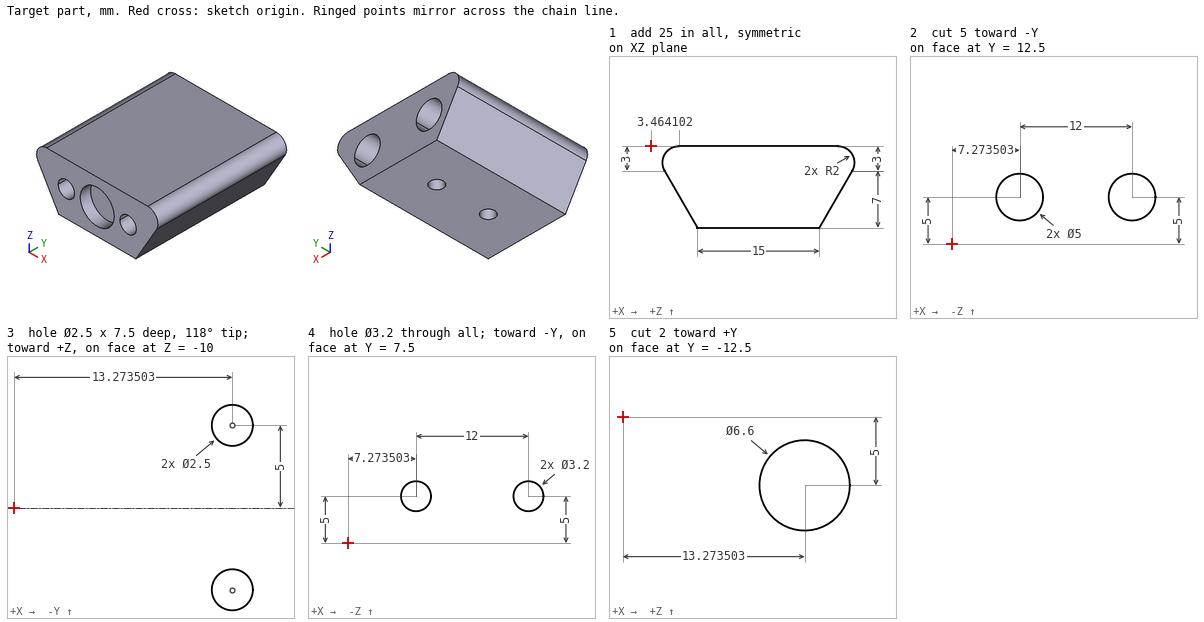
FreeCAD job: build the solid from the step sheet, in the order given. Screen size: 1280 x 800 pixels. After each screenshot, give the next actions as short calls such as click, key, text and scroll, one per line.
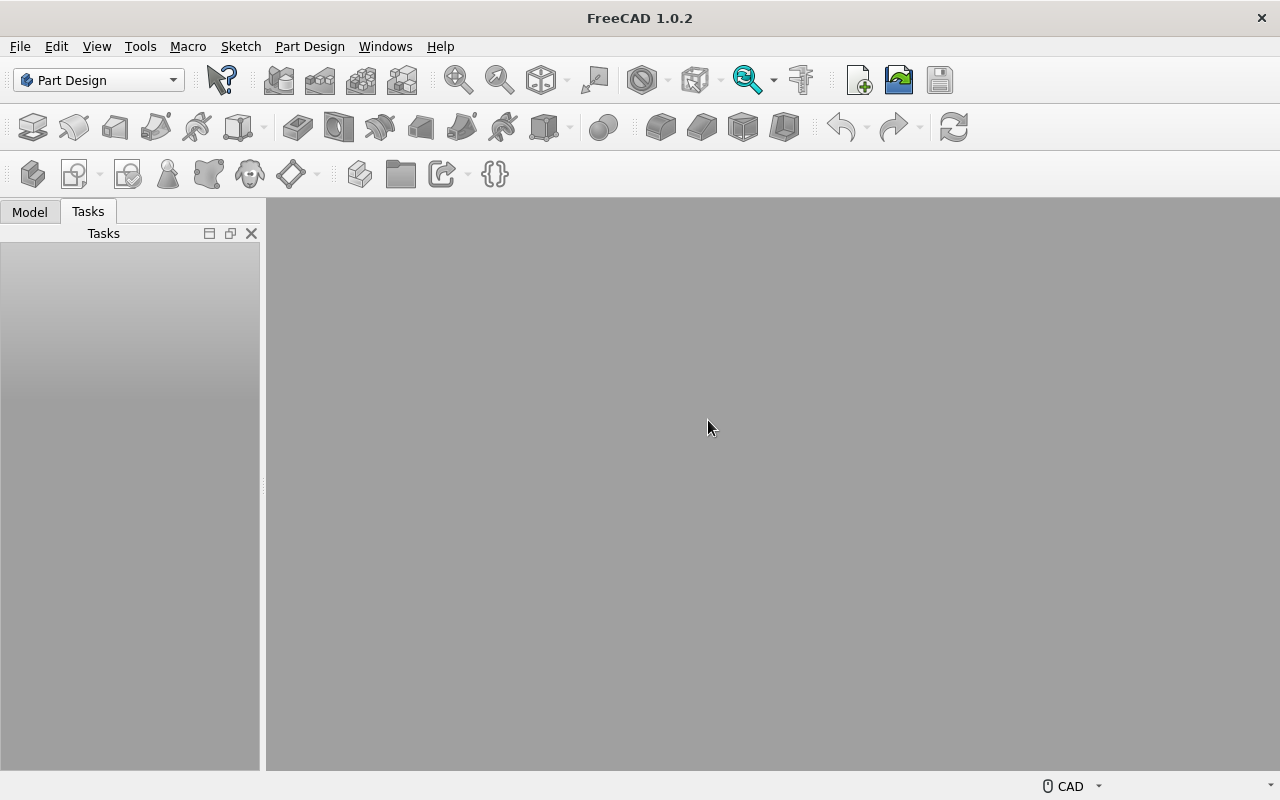
click(858, 80)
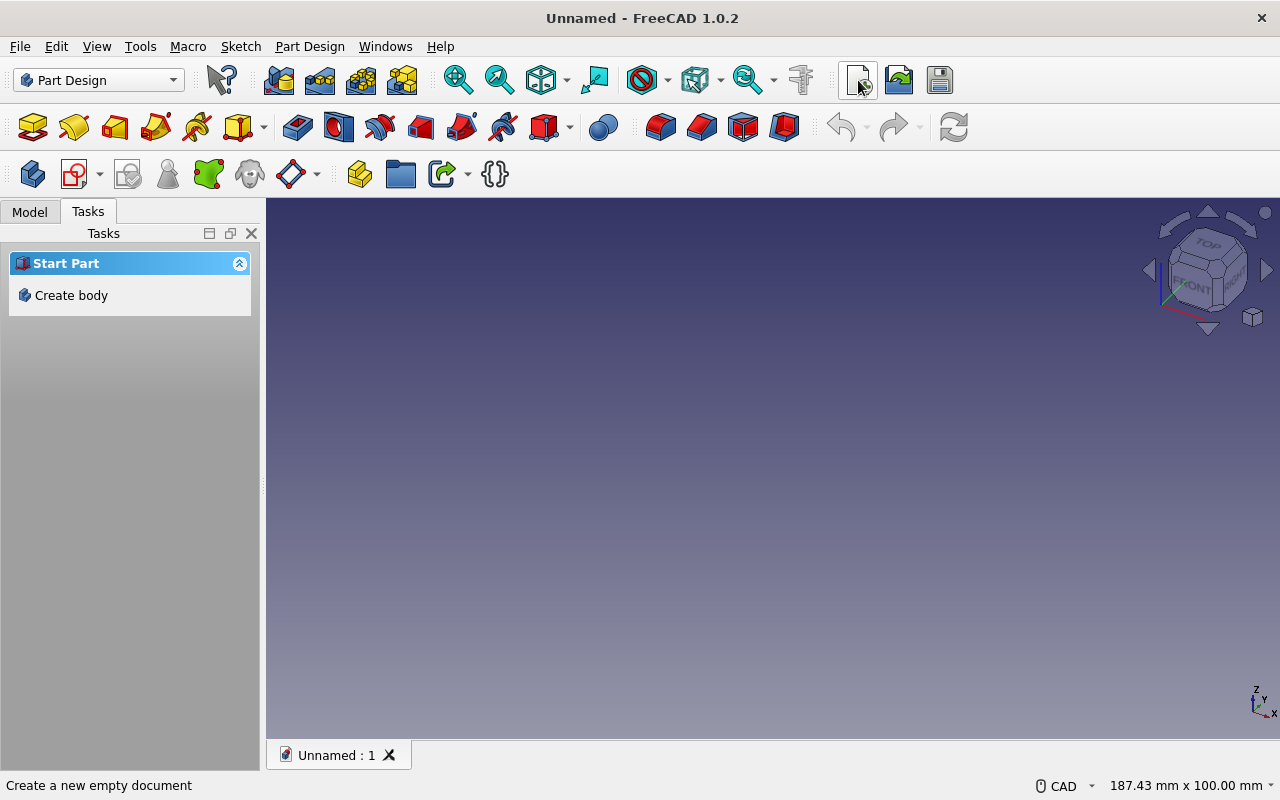
click(74, 174)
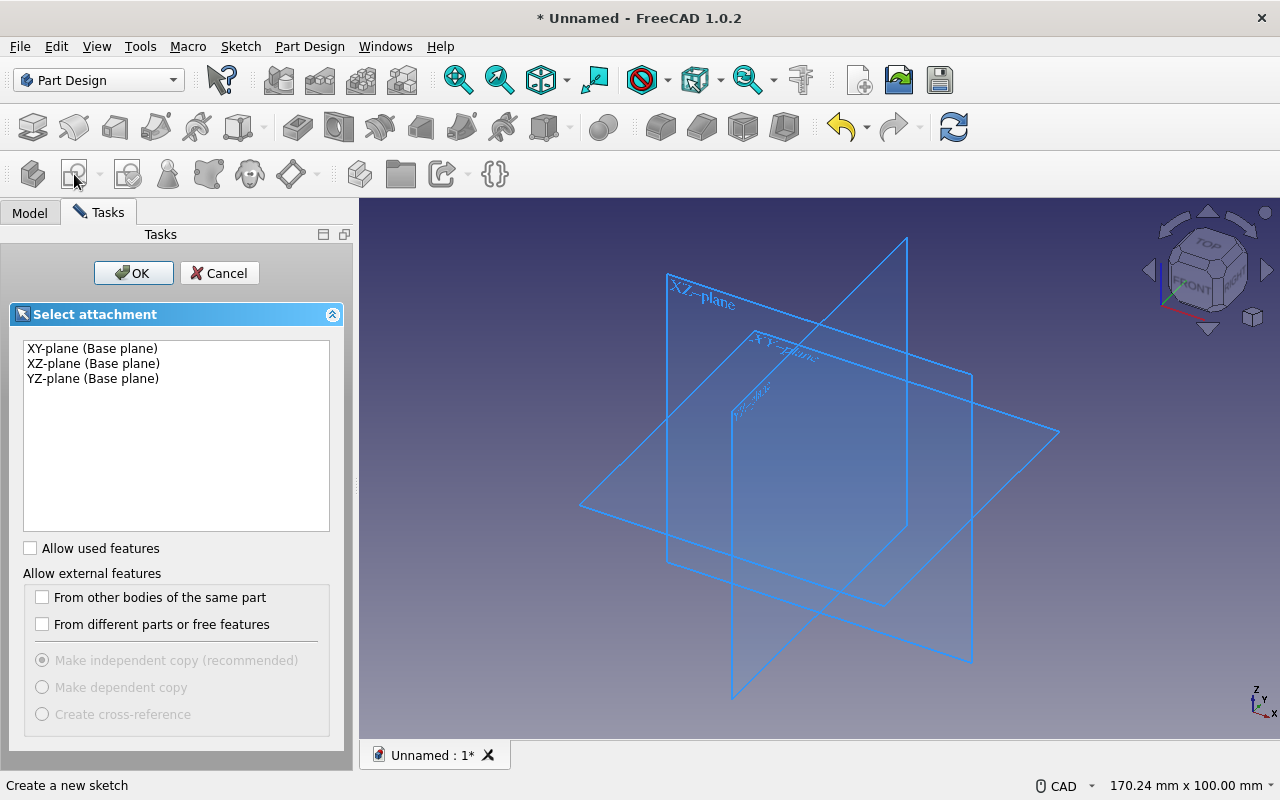
click(84, 364)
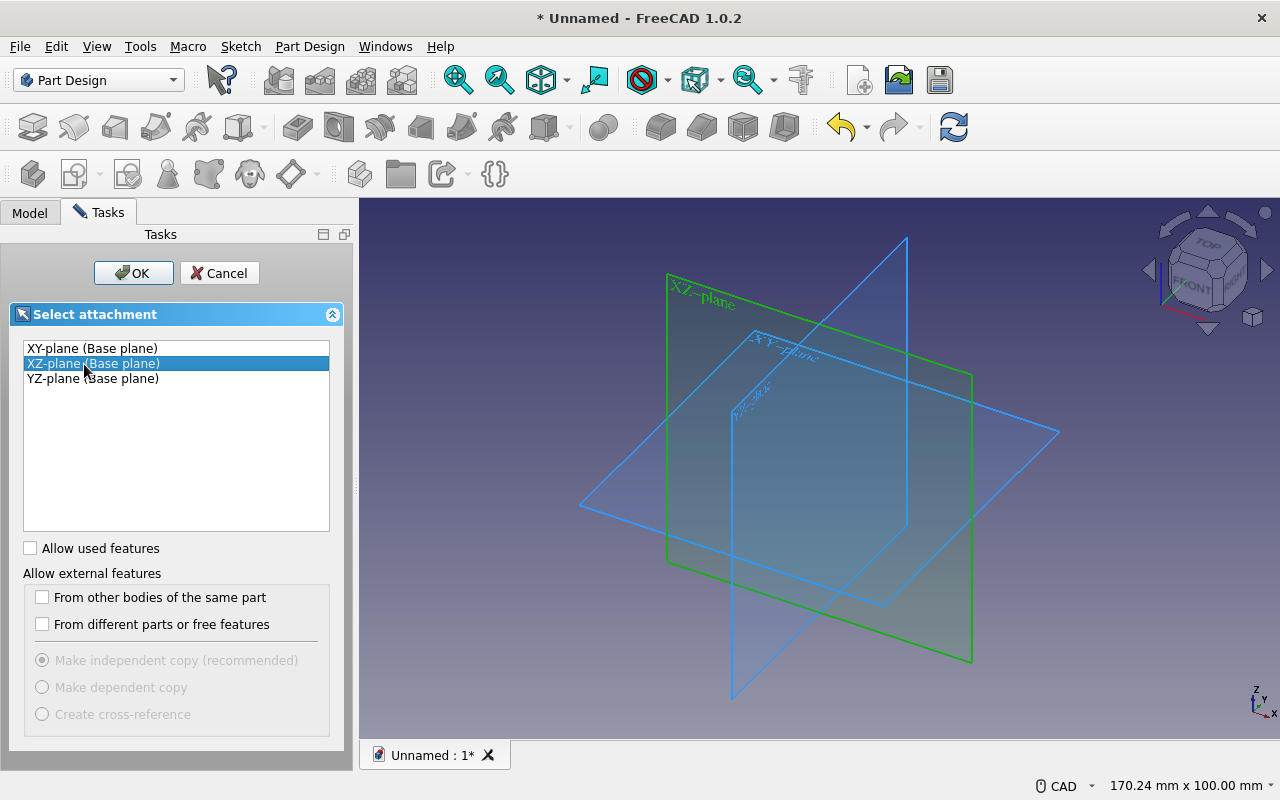
click(134, 273)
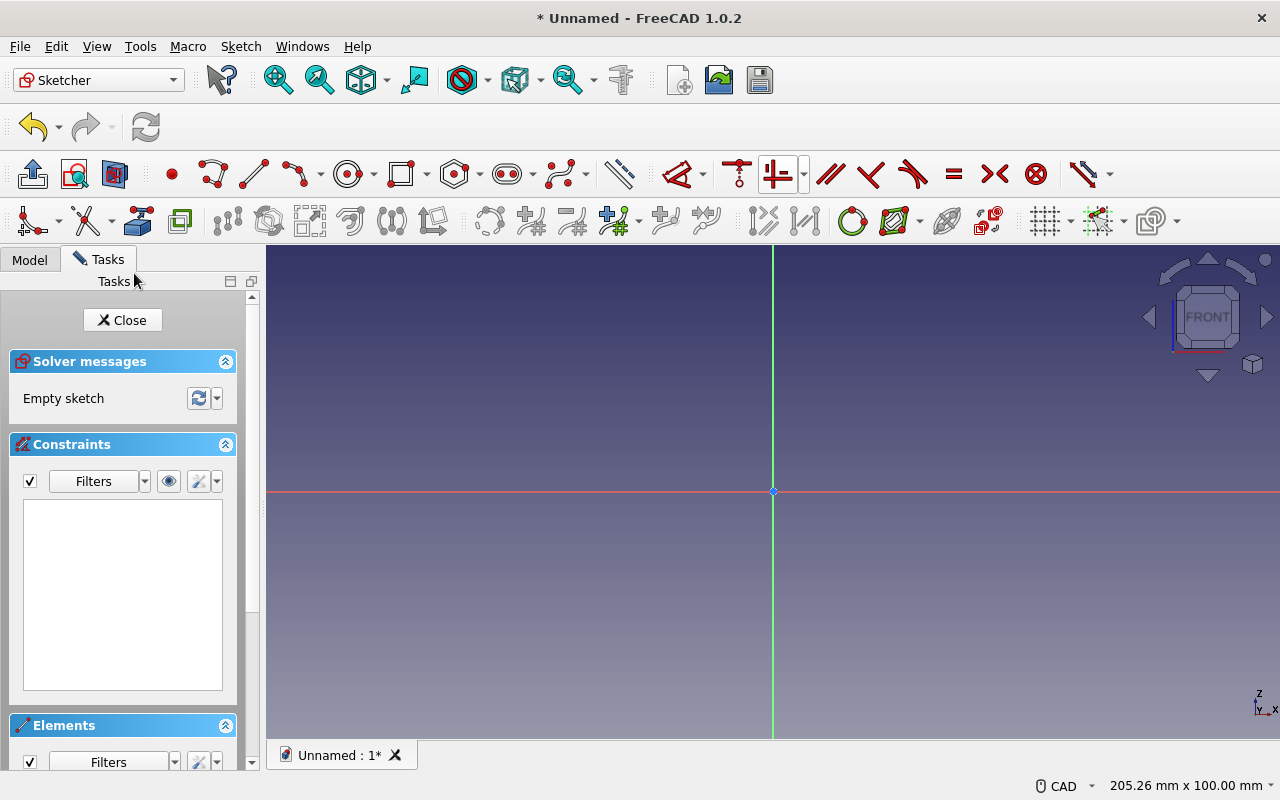
scroll(867, 523, up, 8)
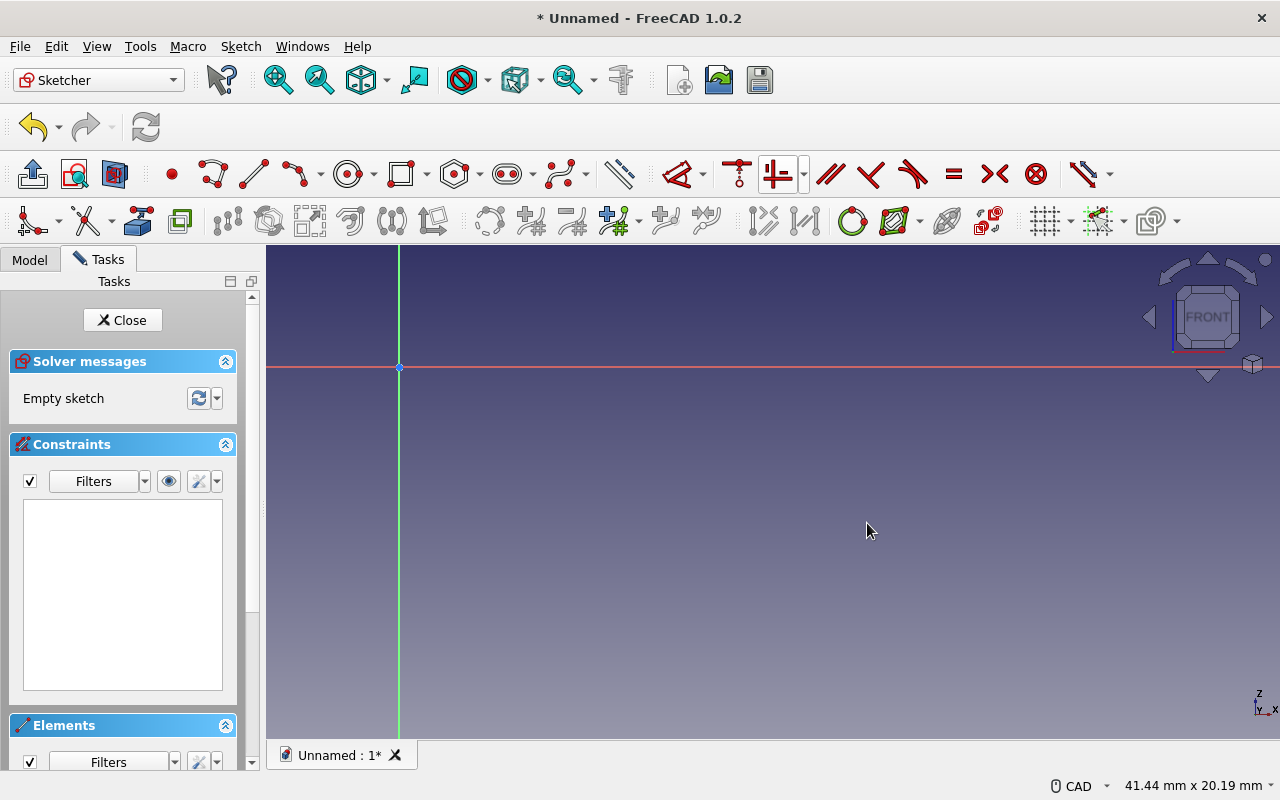
click(254, 174)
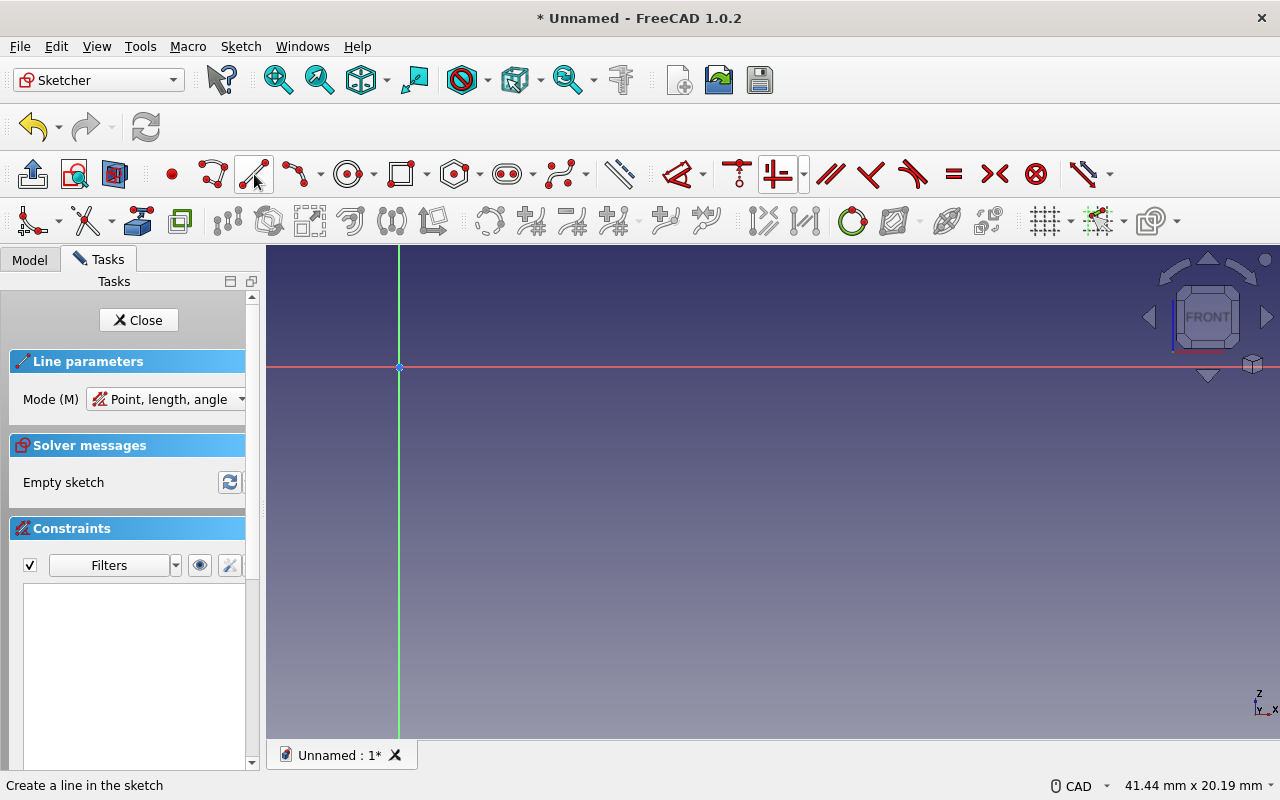
click(484, 367)
click(964, 376)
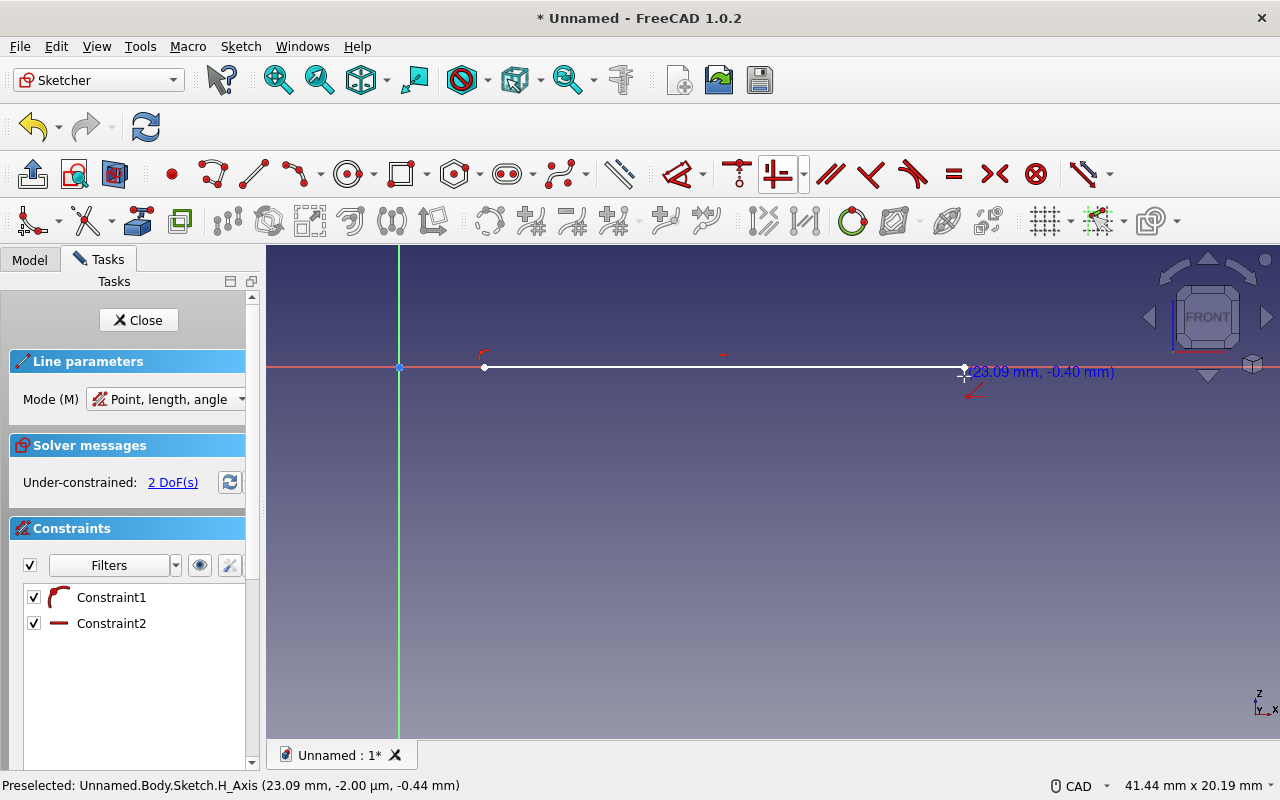
click(213, 174)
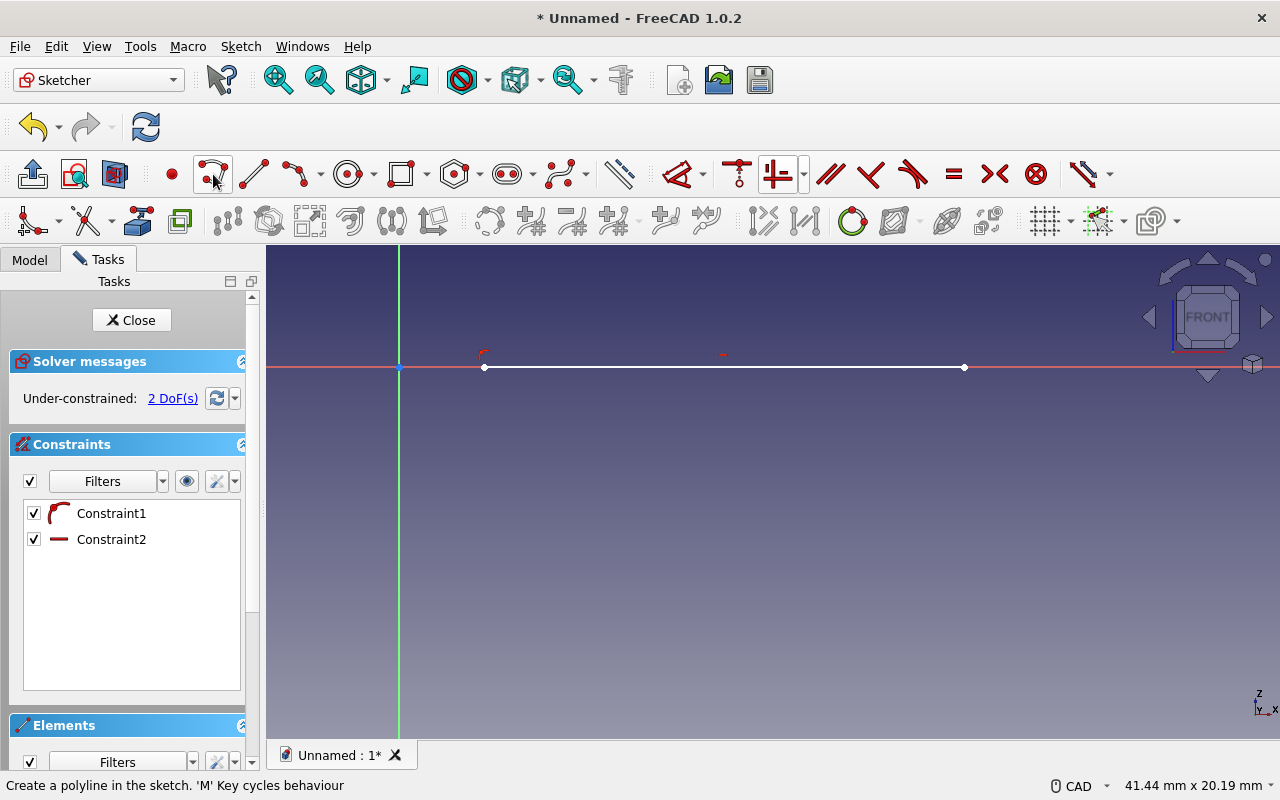
click(1006, 441)
click(907, 612)
click(540, 612)
click(441, 441)
right_click(441, 441)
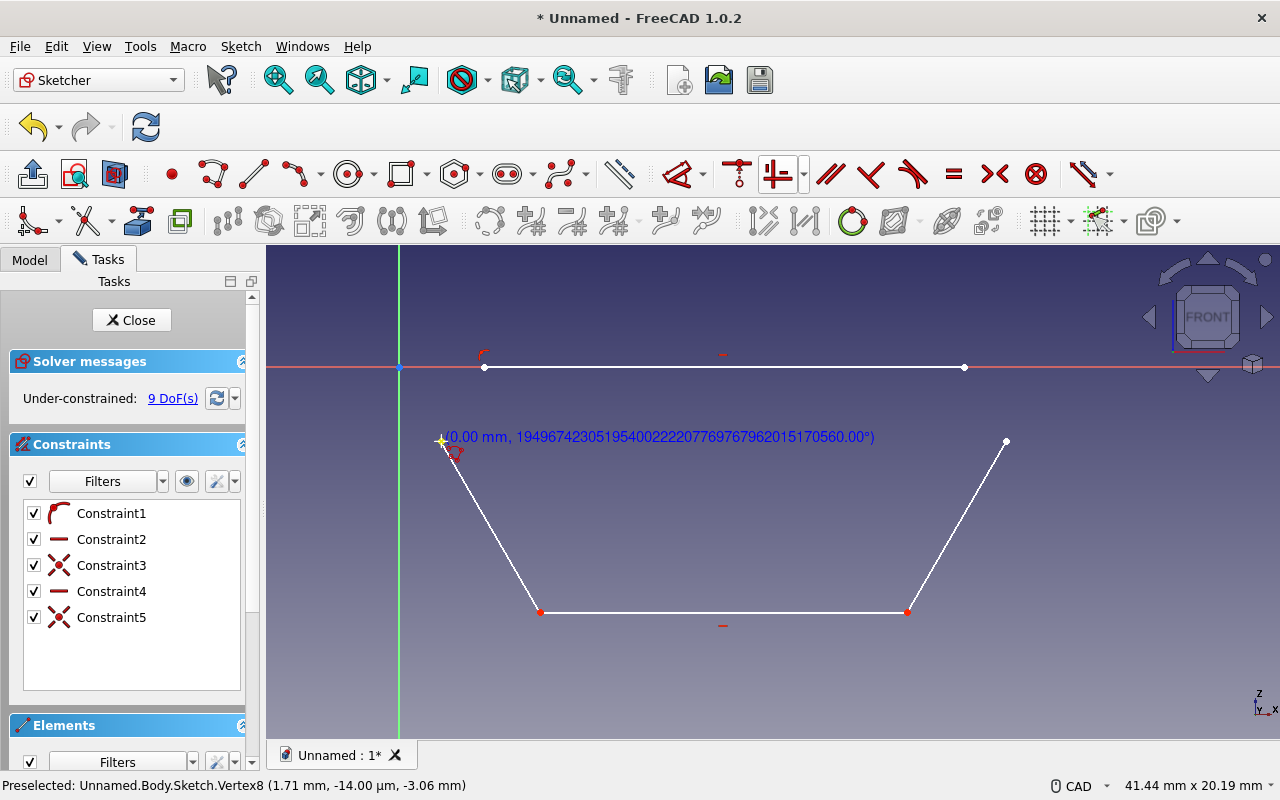
key(g)
key(3)
key(a)